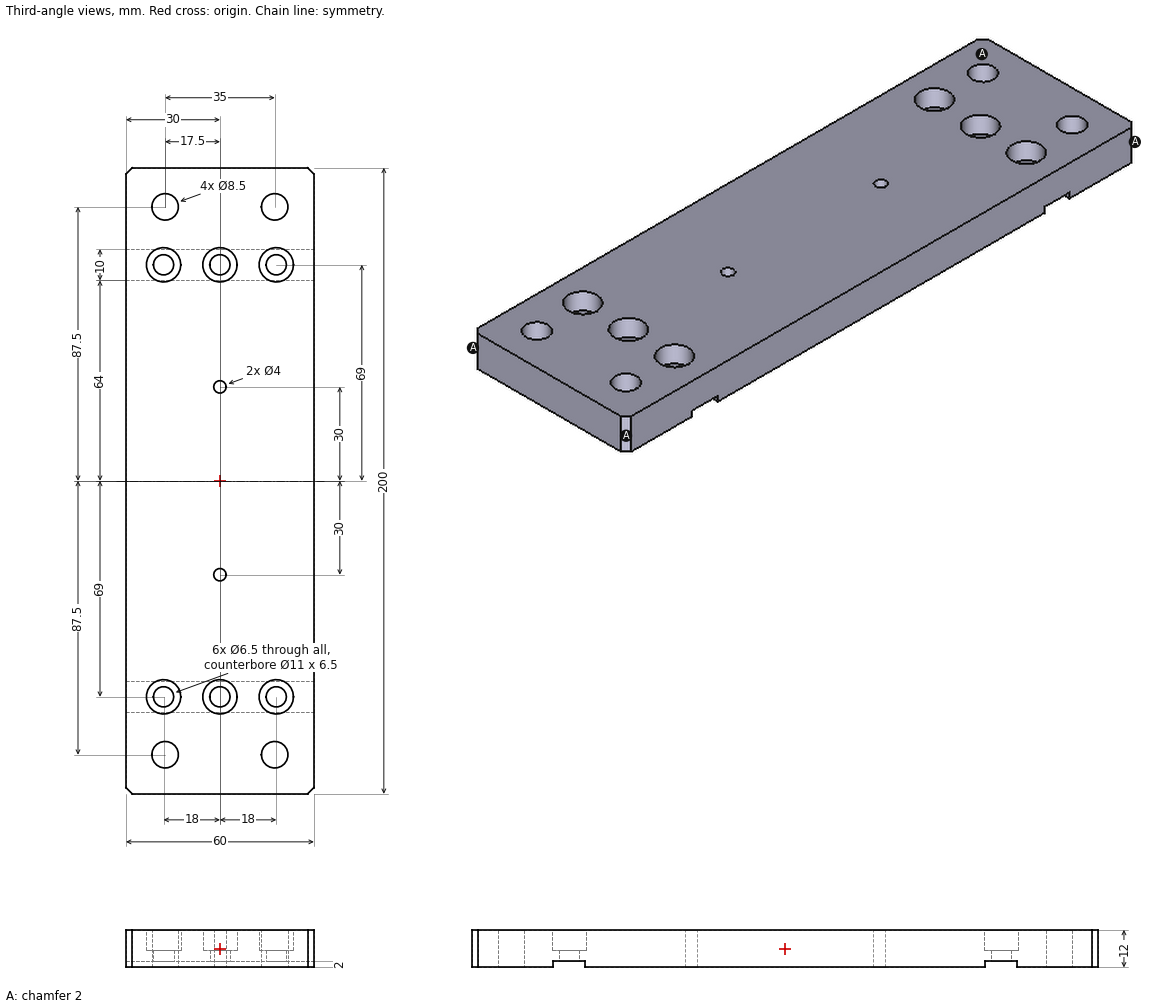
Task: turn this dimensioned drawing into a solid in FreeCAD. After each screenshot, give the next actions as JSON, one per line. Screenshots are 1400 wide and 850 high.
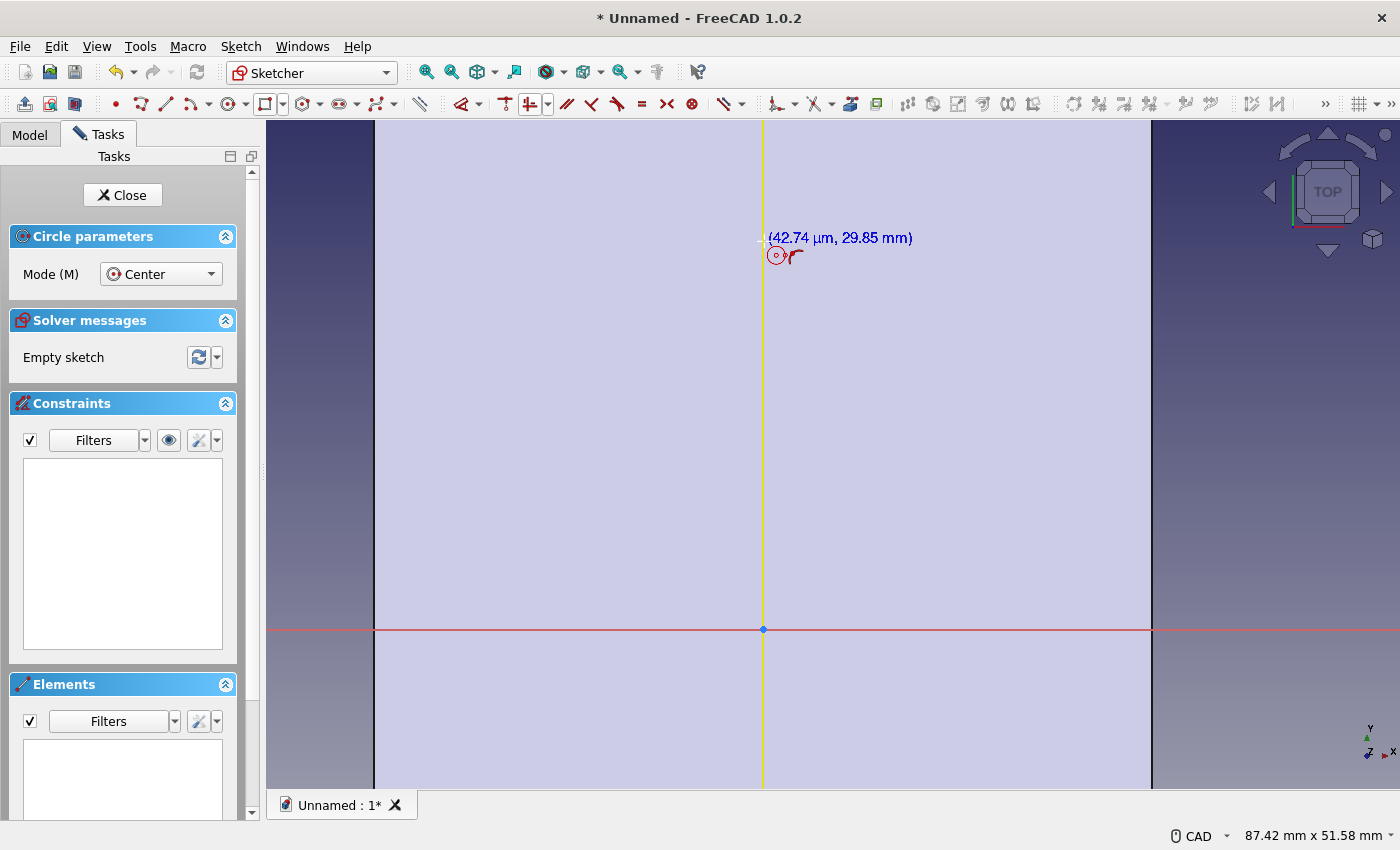
{"action": "left_click", "coordinate": [763, 241]}
{"action": "left_click", "coordinate": [781, 222]}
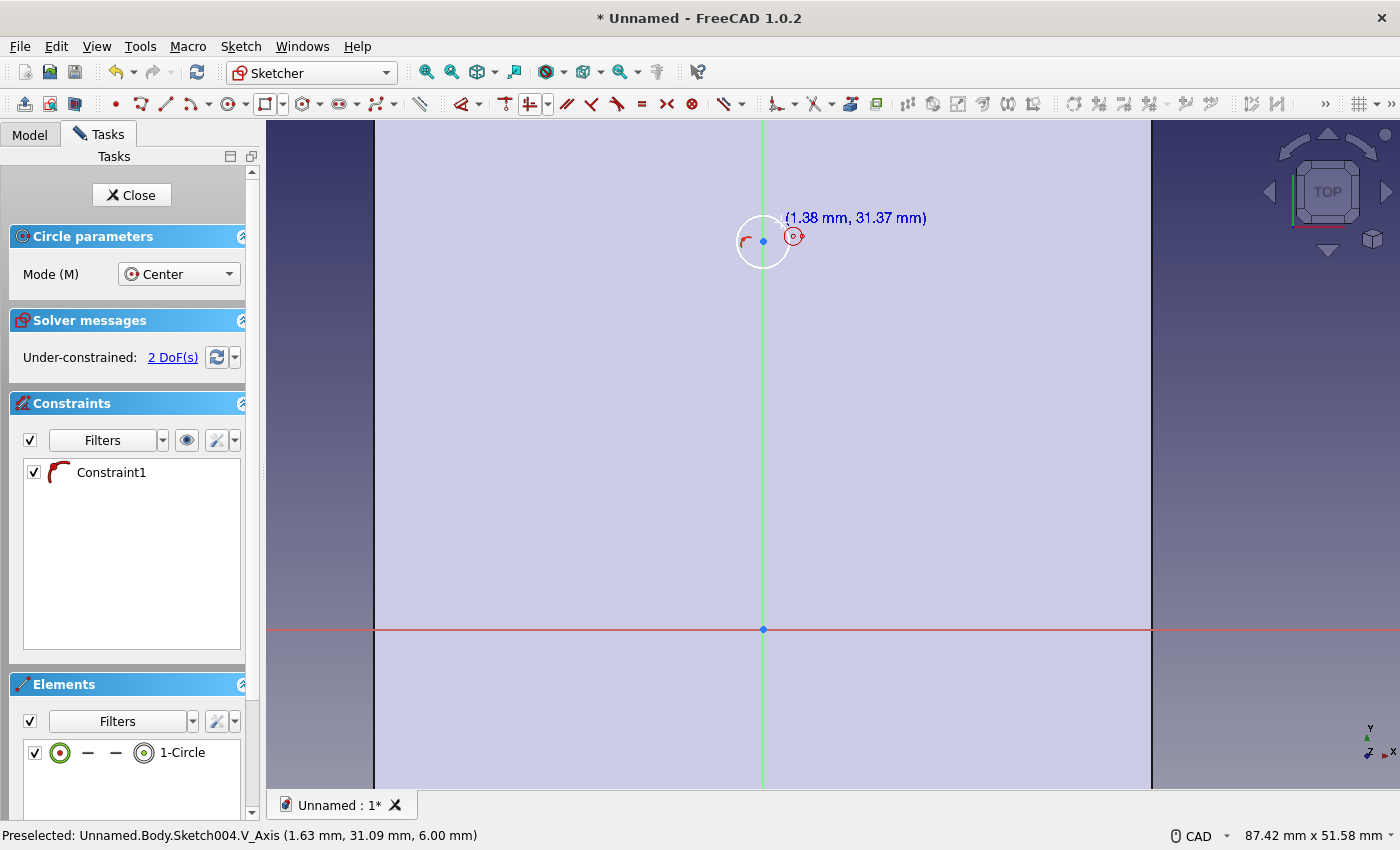
{"action": "scroll", "coordinate": [766, 241], "scroll_direction": "down", "scroll_amount": 3}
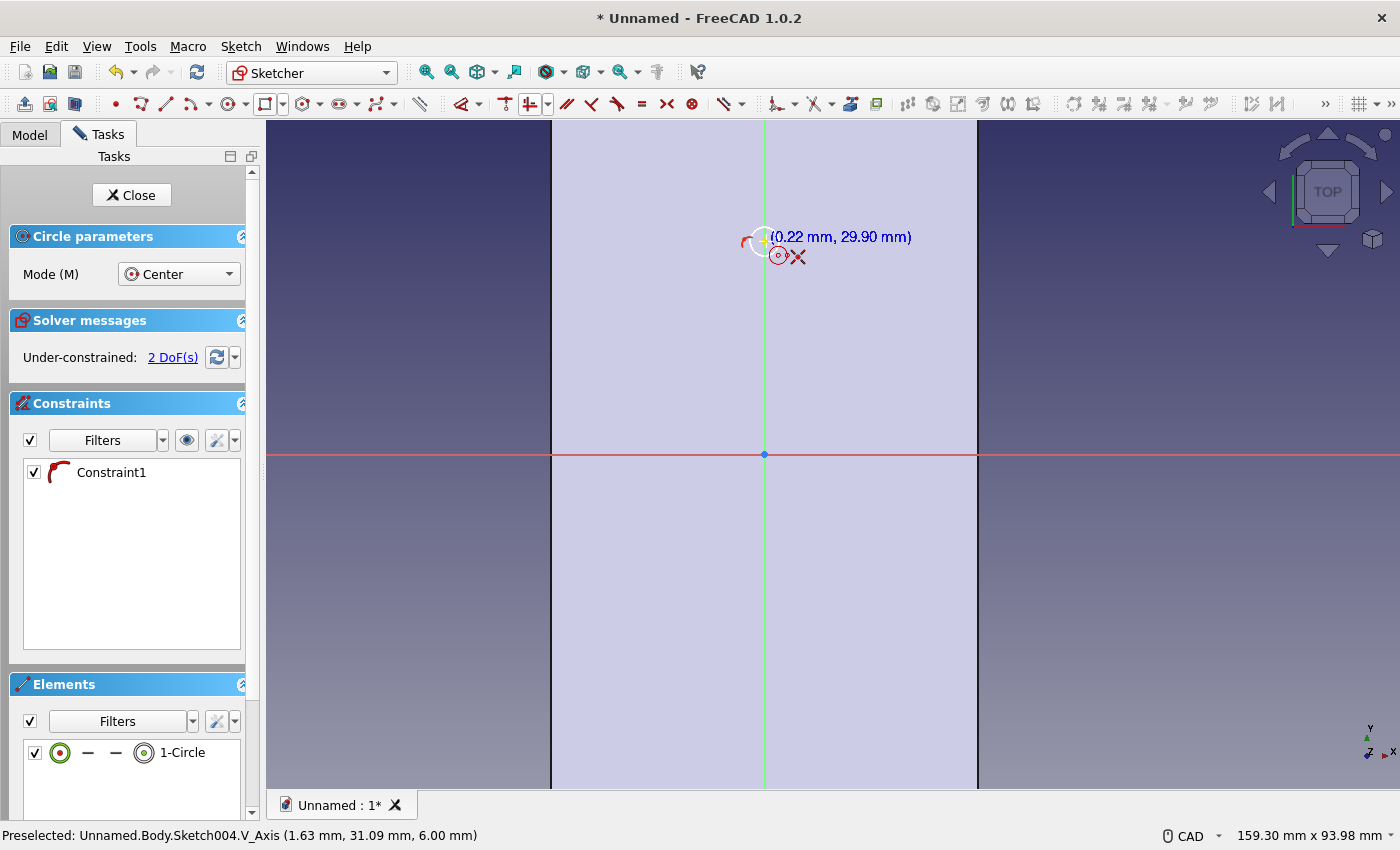
{"action": "scroll", "coordinate": [765, 668], "scroll_direction": "up", "scroll_amount": 3}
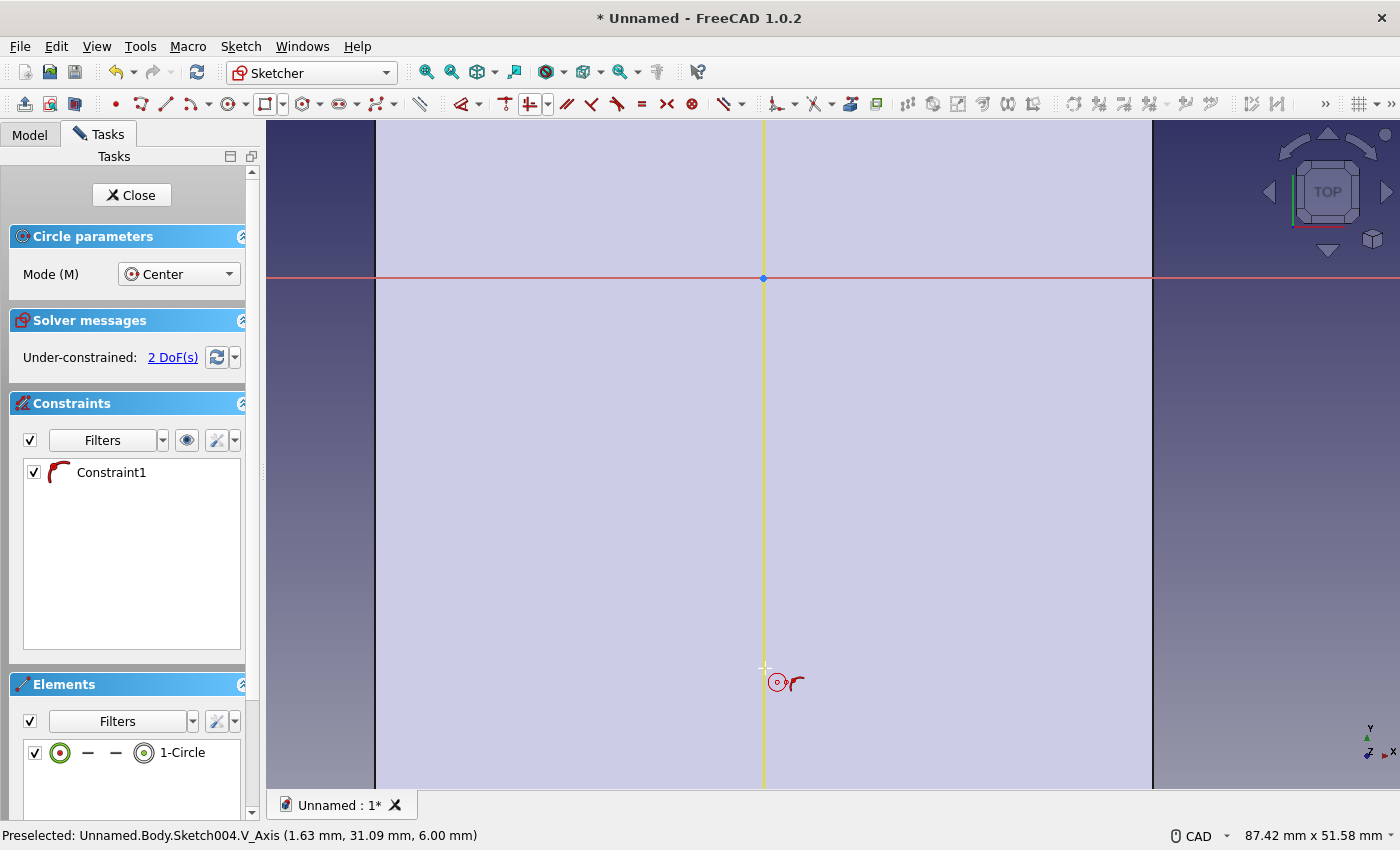
{"action": "left_click", "coordinate": [764, 667]}
{"action": "left_click", "coordinate": [782, 649]}
{"action": "key", "text": "Escape"}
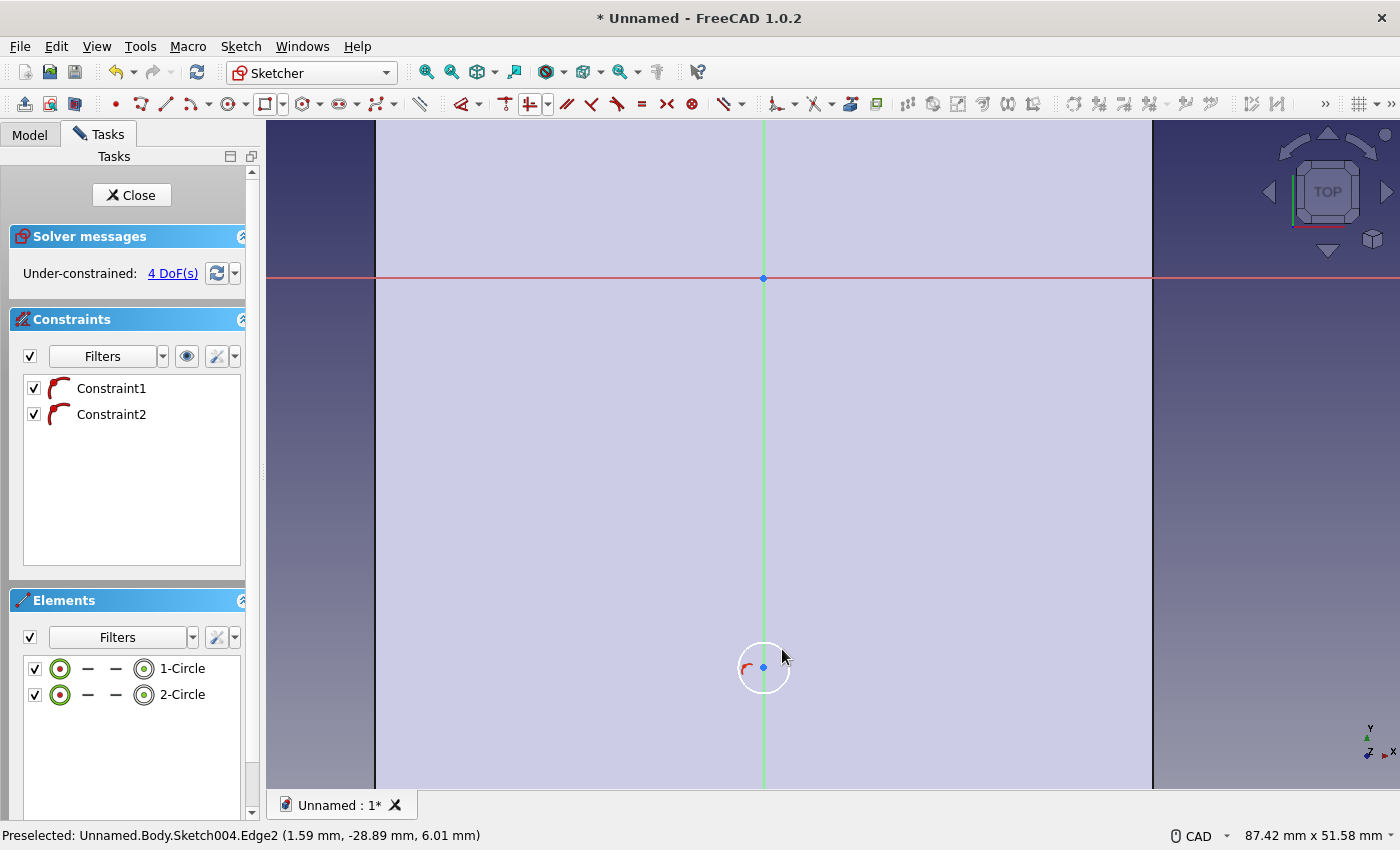
{"action": "scroll", "coordinate": [765, 669], "scroll_direction": "down", "scroll_amount": 3}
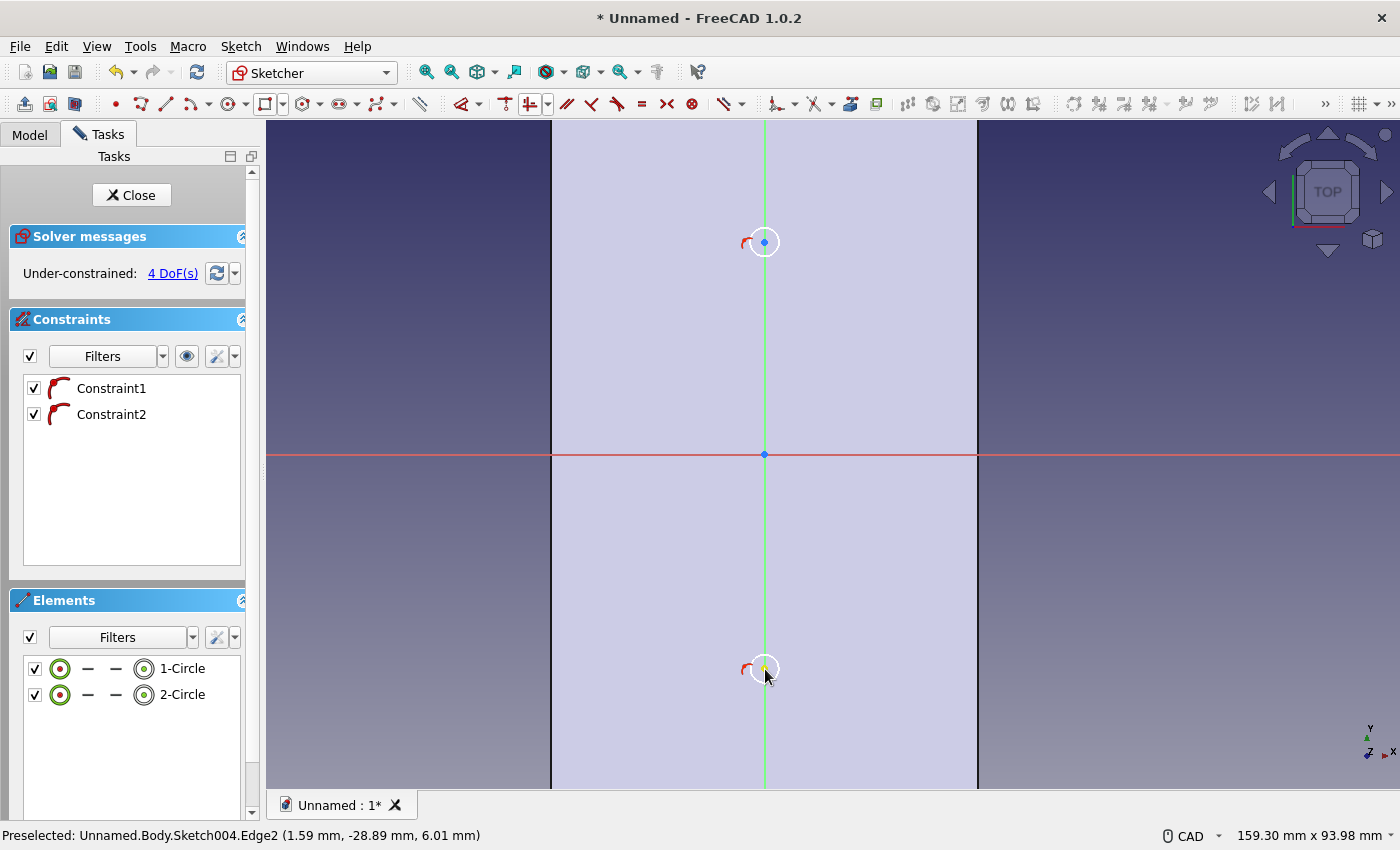
{"action": "scroll", "coordinate": [775, 232], "scroll_direction": "up", "scroll_amount": 2}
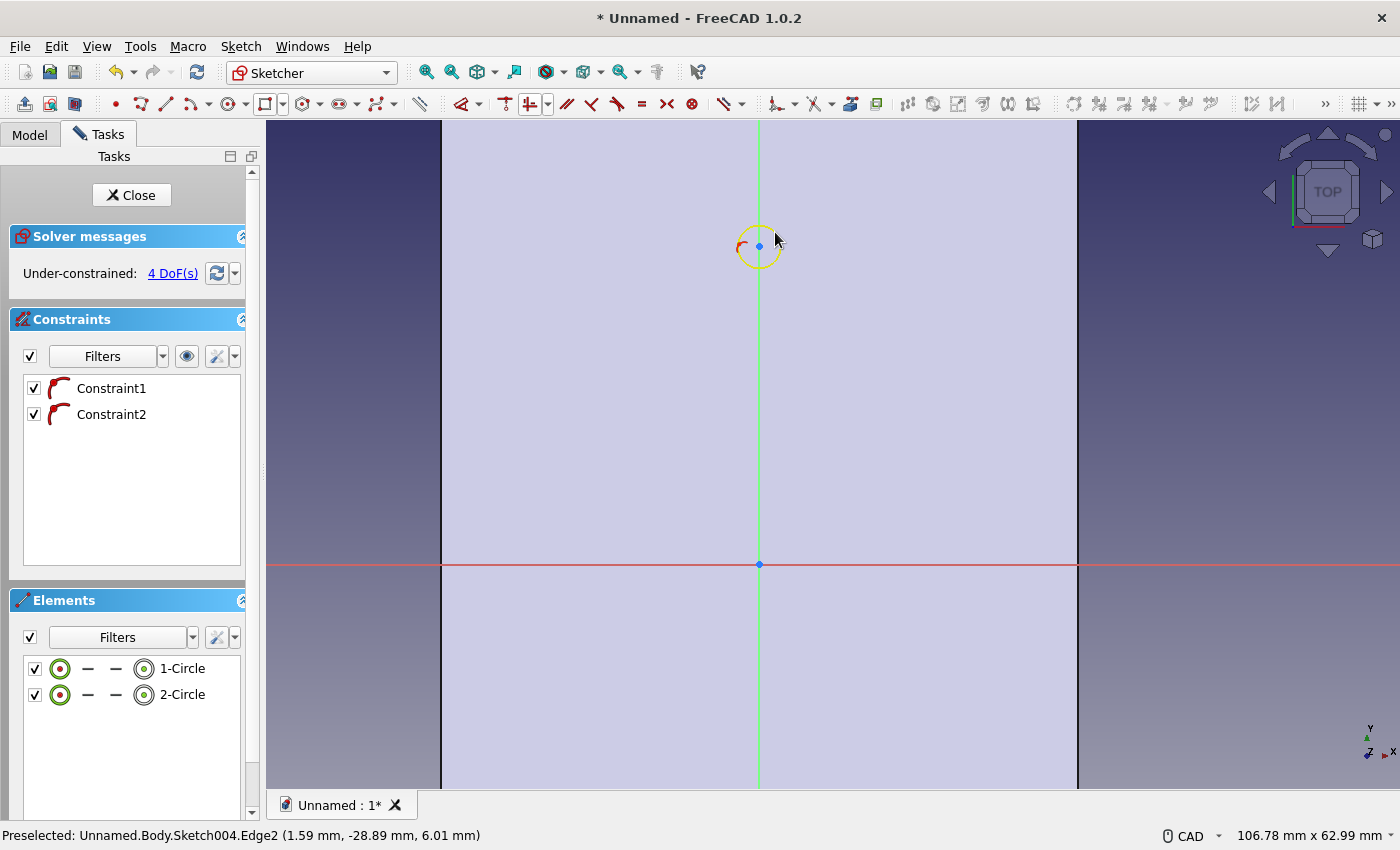
{"action": "left_click", "coordinate": [774, 232]}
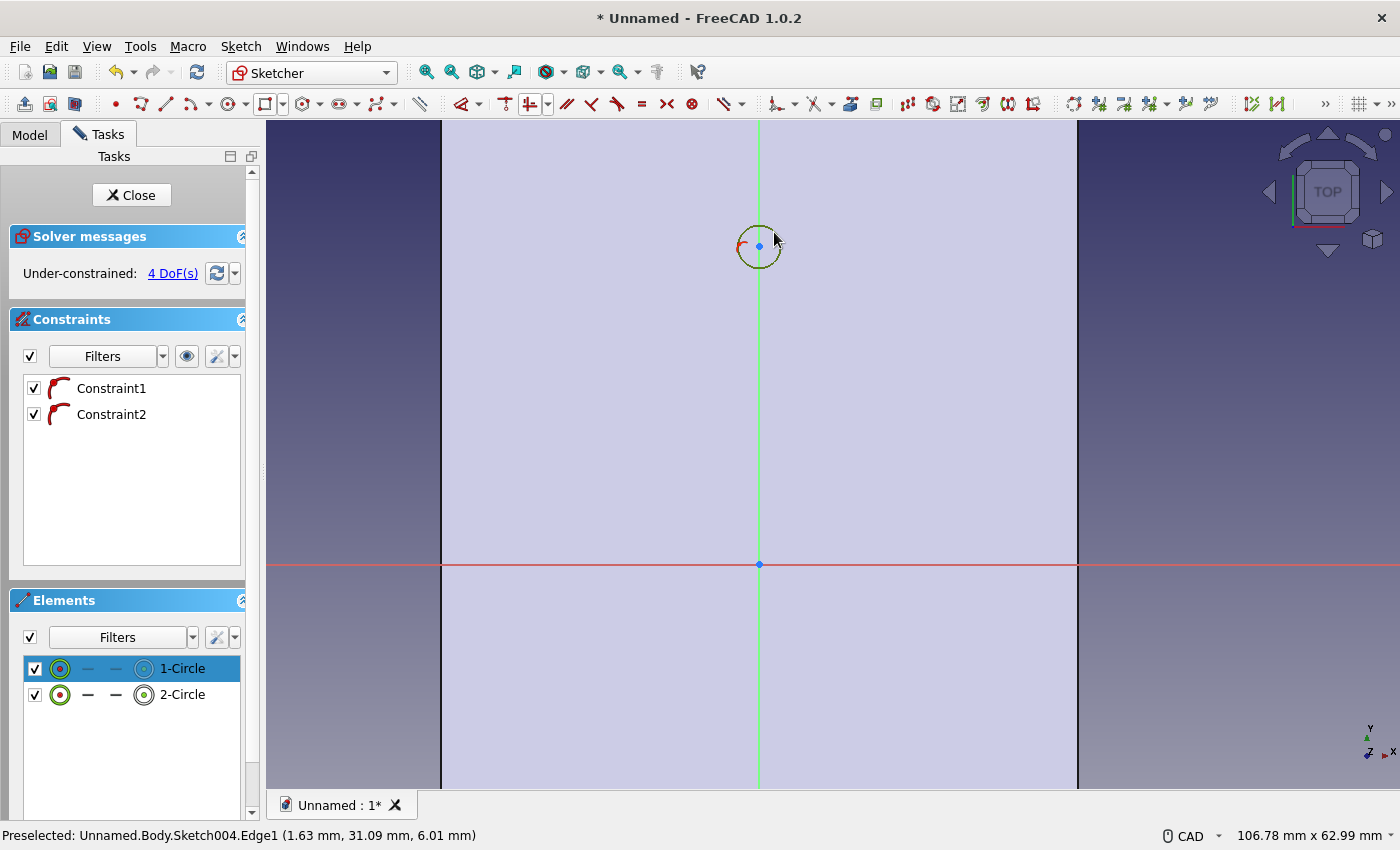
{"action": "scroll", "coordinate": [775, 231], "scroll_direction": "down", "scroll_amount": 2}